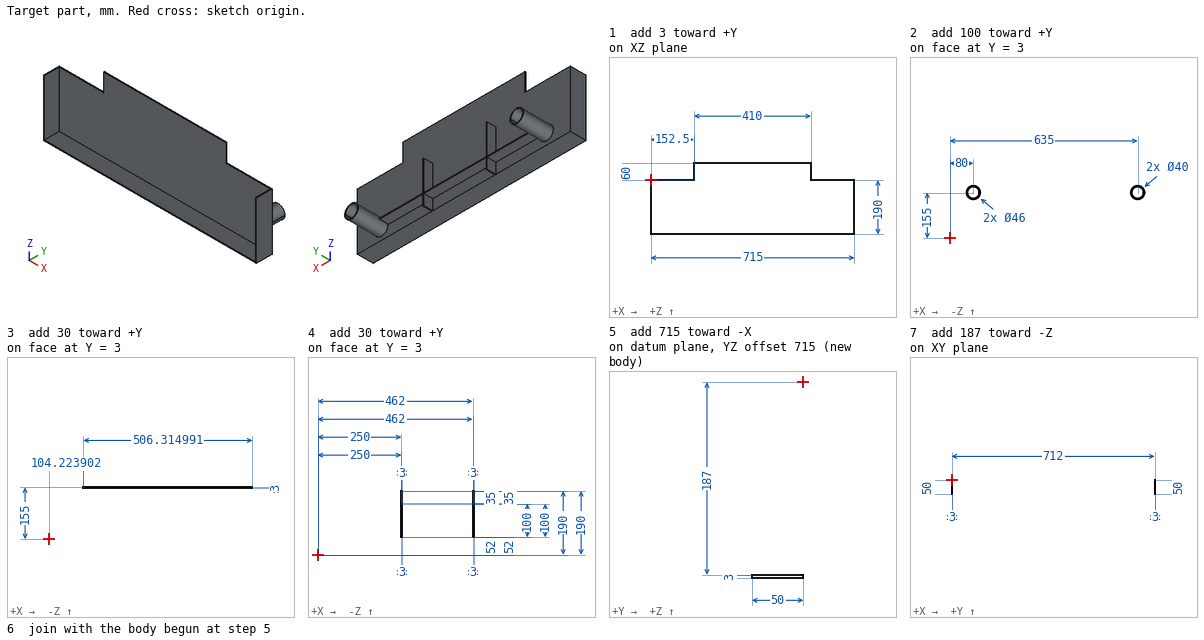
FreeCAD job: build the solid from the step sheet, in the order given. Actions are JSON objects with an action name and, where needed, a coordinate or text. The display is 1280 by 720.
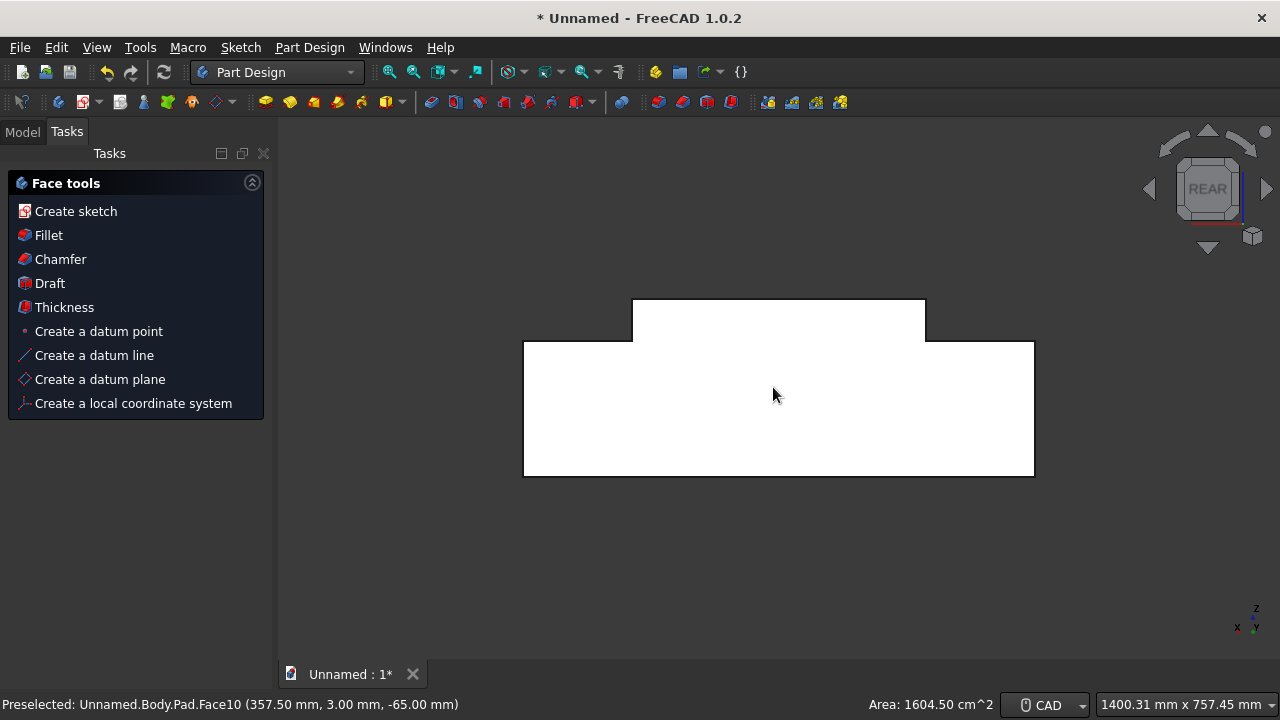
{"action": "left_click", "coordinate": [84, 102]}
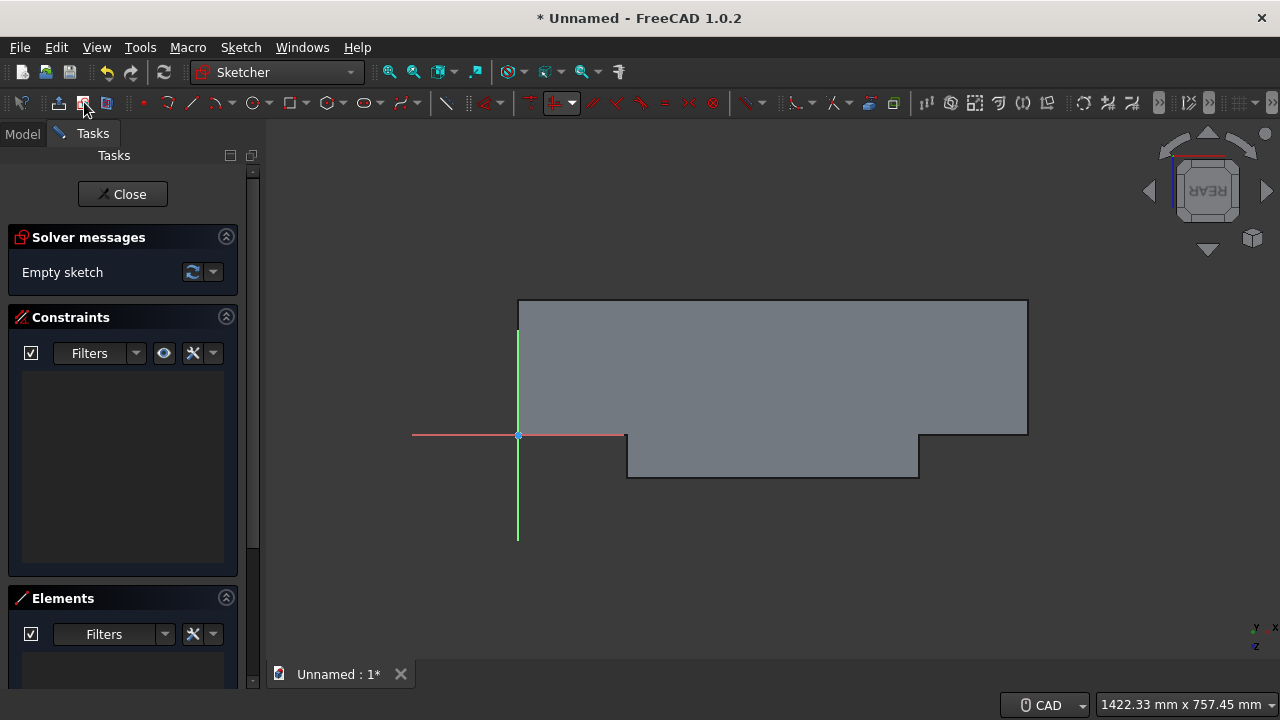
{"action": "key", "text": "g c"}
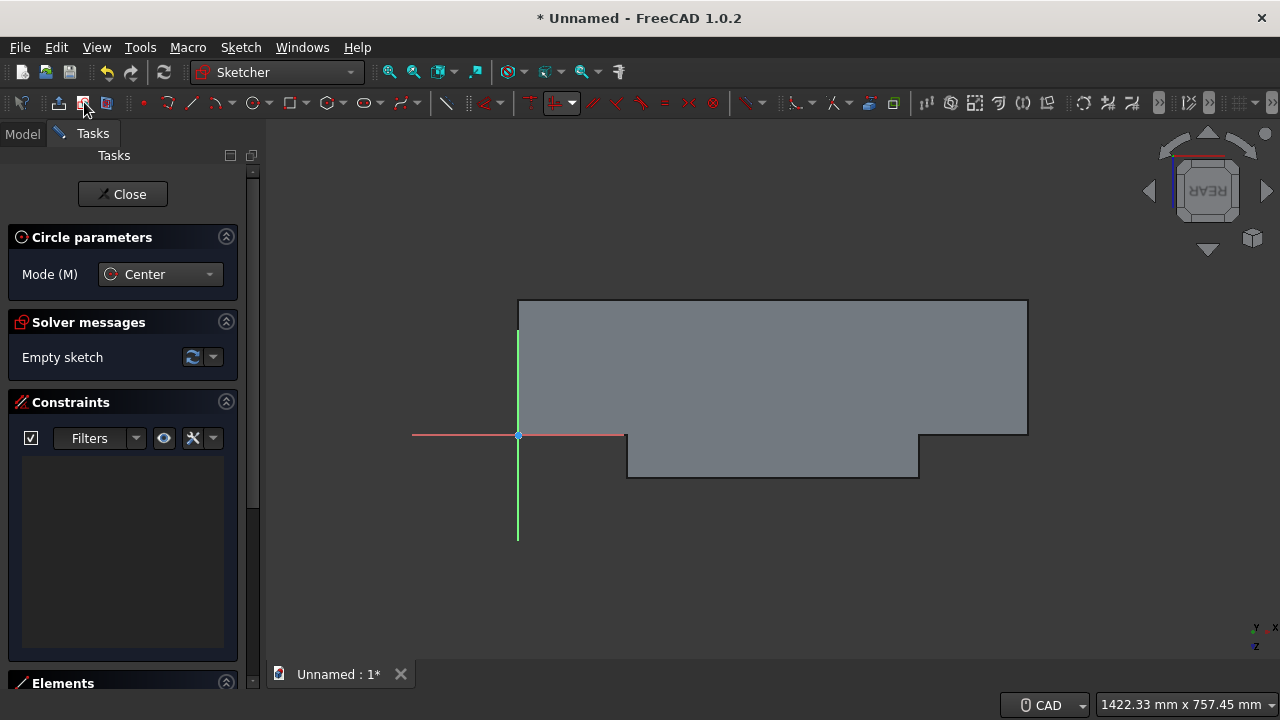
{"action": "scroll", "coordinate": [575, 325], "scroll_direction": "up", "scroll_amount": 2}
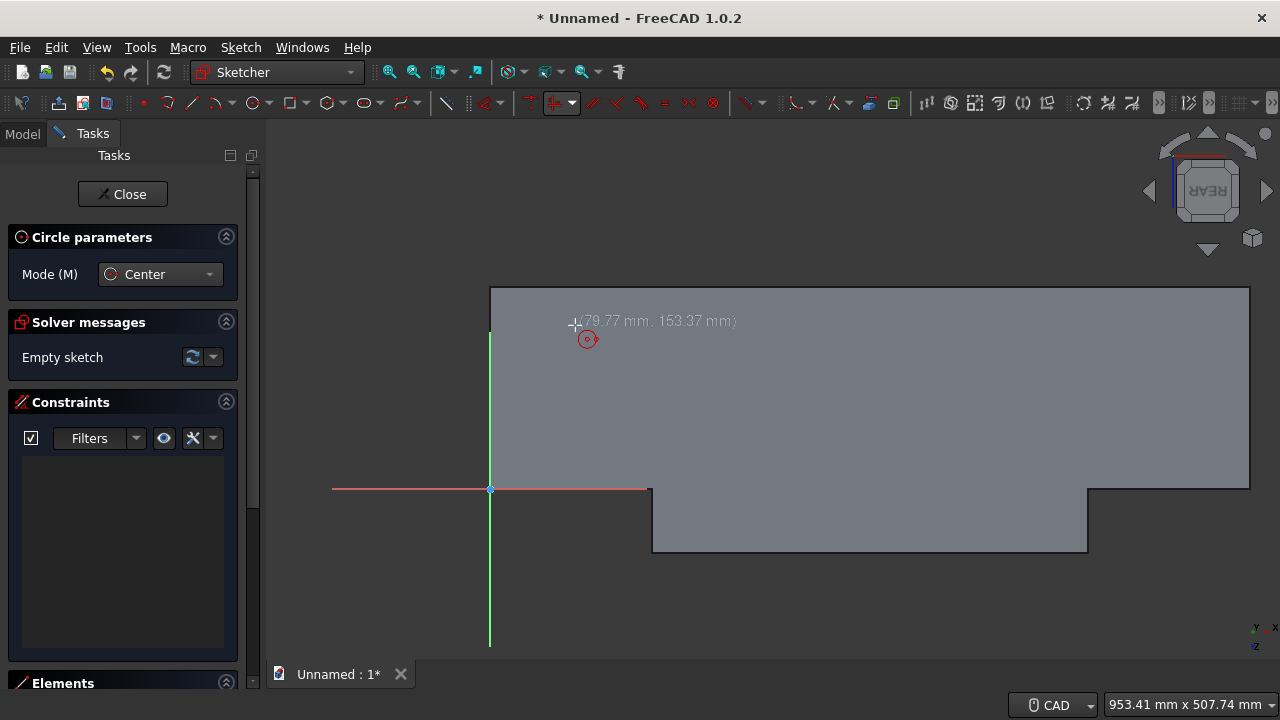
{"action": "left_click", "coordinate": [575, 325]}
{"action": "mouse_move", "coordinate": [592, 307]}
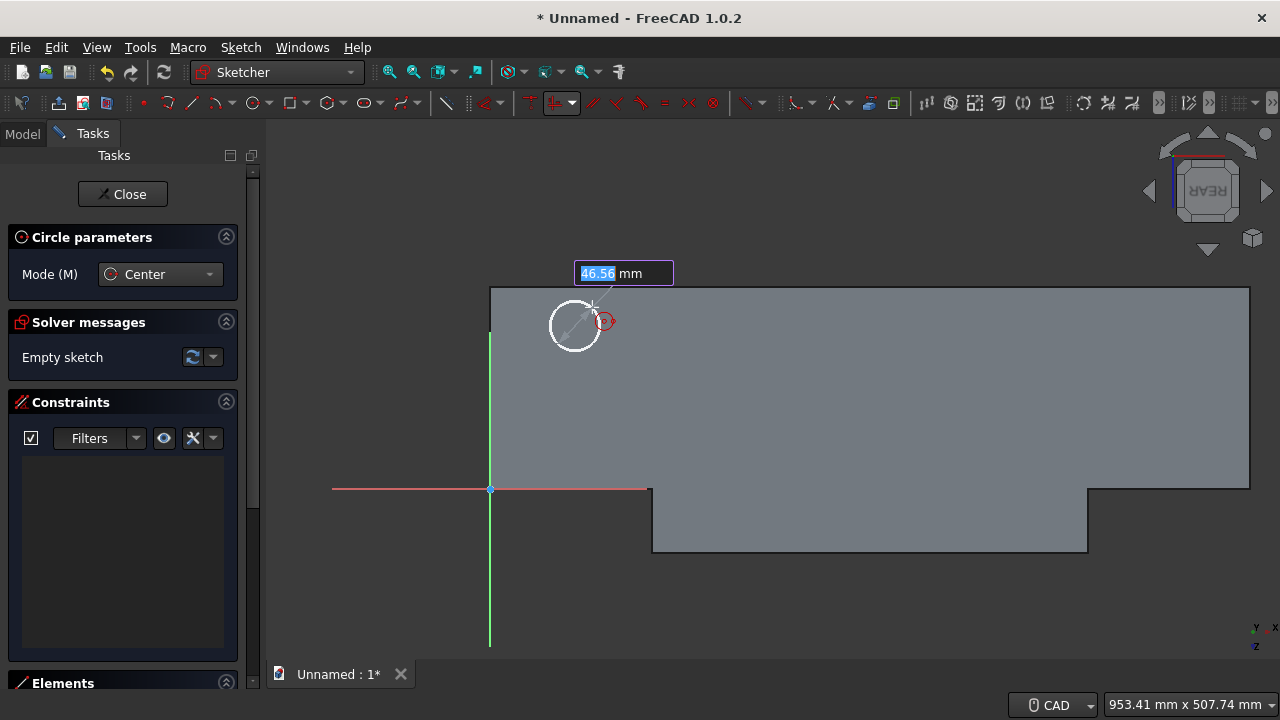
{"action": "type", "text": "46"}
{"action": "key", "text": "Return"}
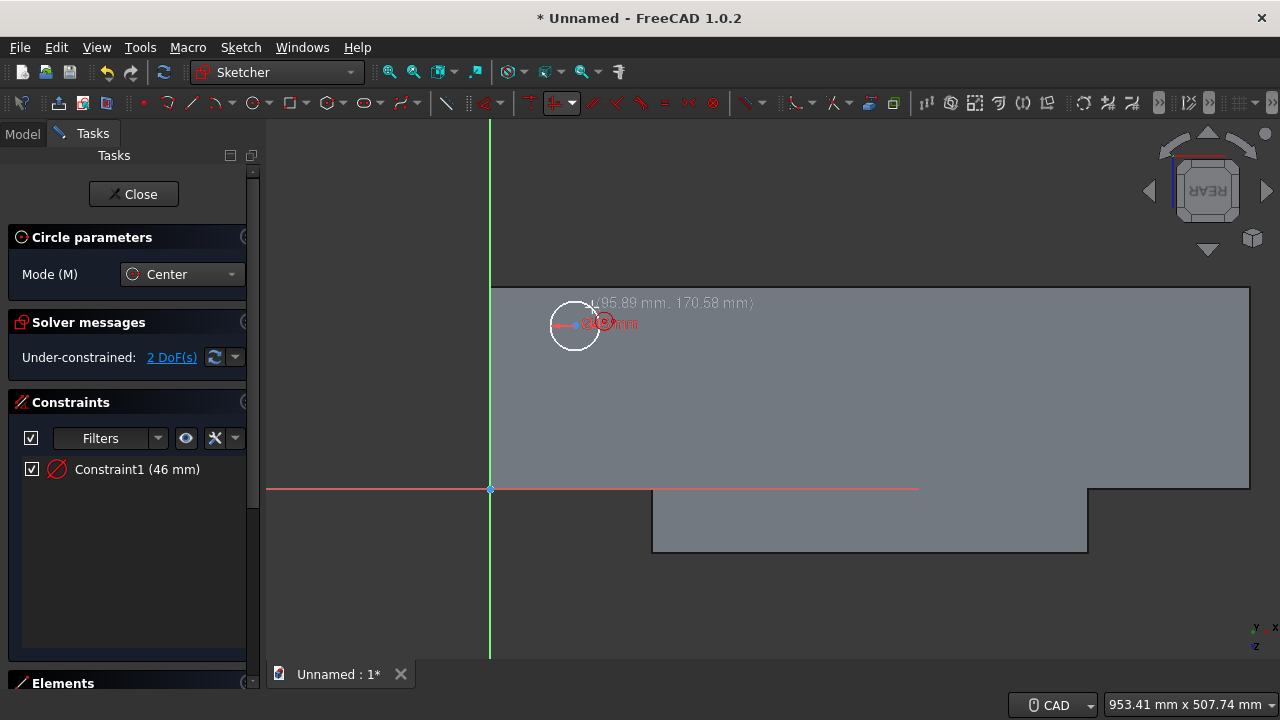
{"action": "scroll", "coordinate": [294, 363], "scroll_direction": "down", "scroll_amount": 1}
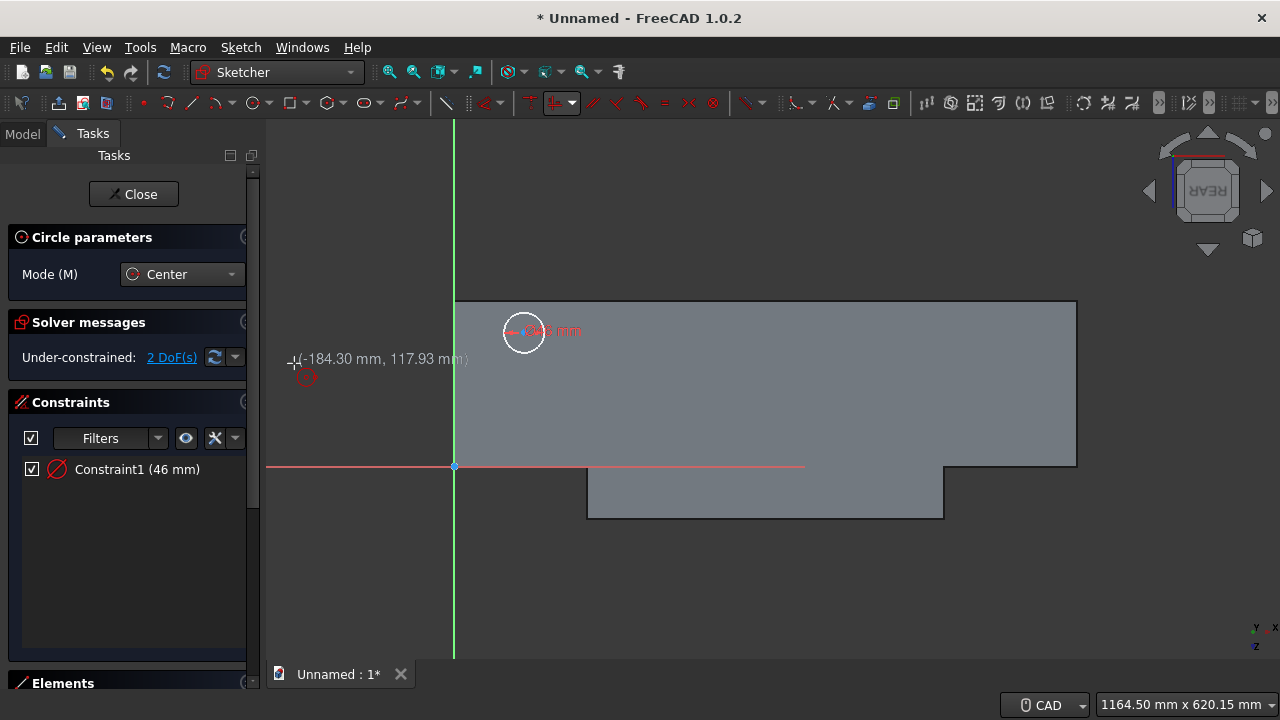
{"action": "left_click", "coordinate": [1007, 332]}
{"action": "mouse_move", "coordinate": [1022, 317]}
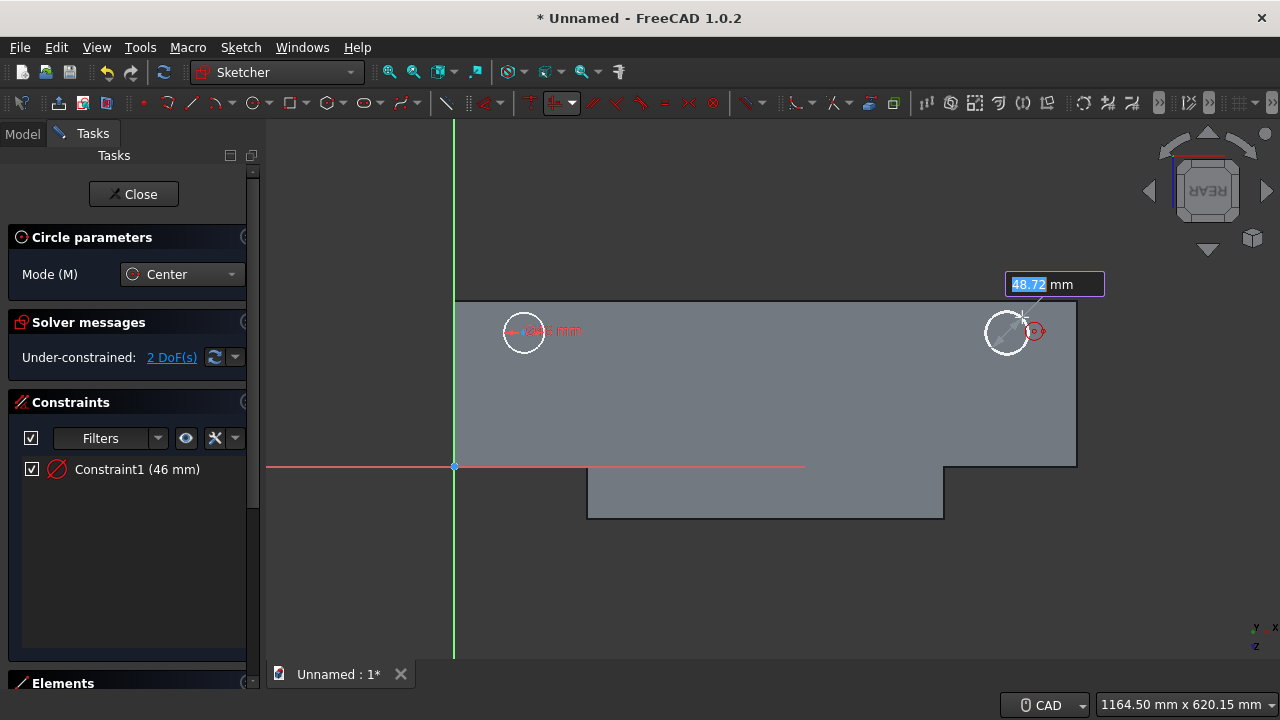
{"action": "type", "text": "46"}
{"action": "key", "text": "Return"}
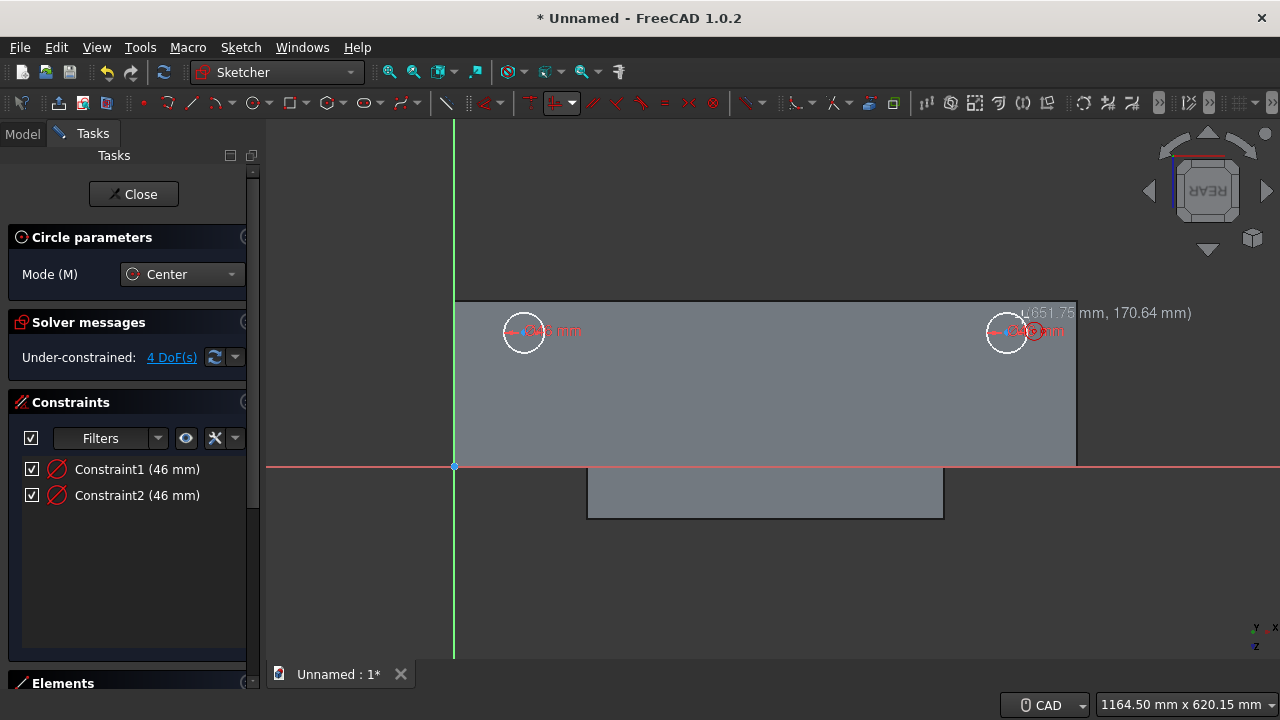
{"action": "scroll", "coordinate": [524, 332], "scroll_direction": "up", "scroll_amount": 2}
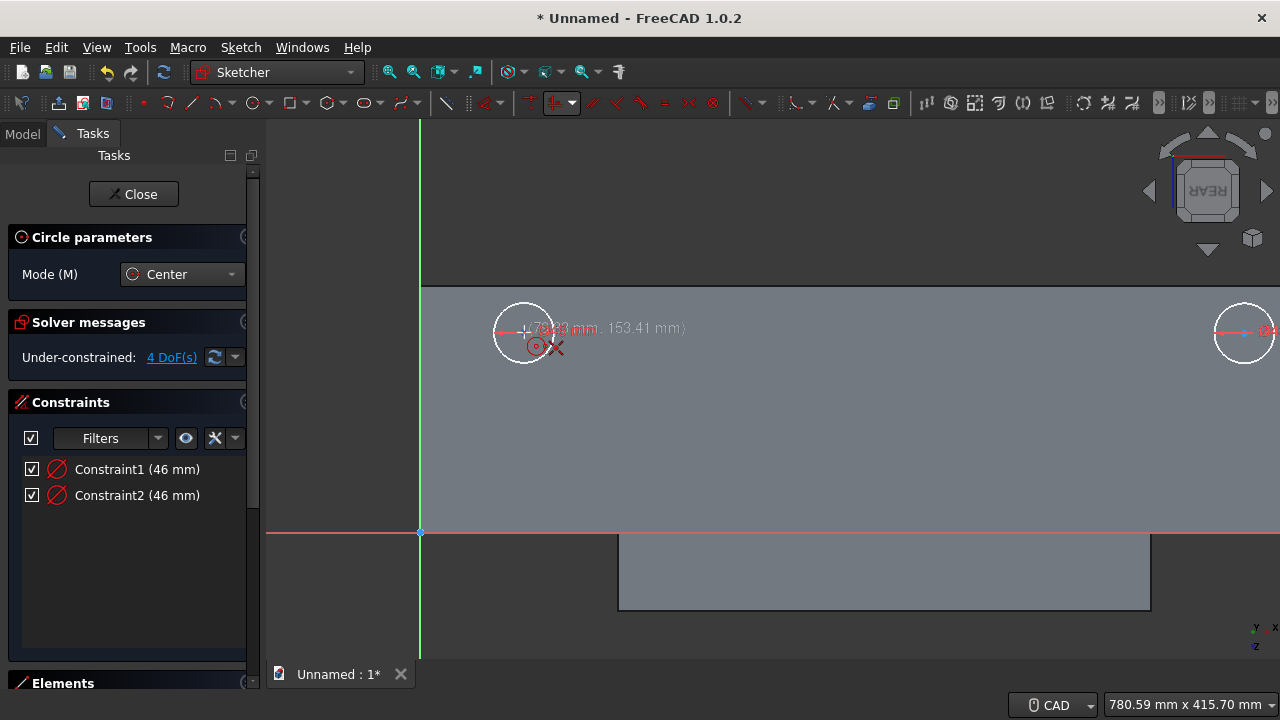
{"action": "left_click", "coordinate": [524, 333]}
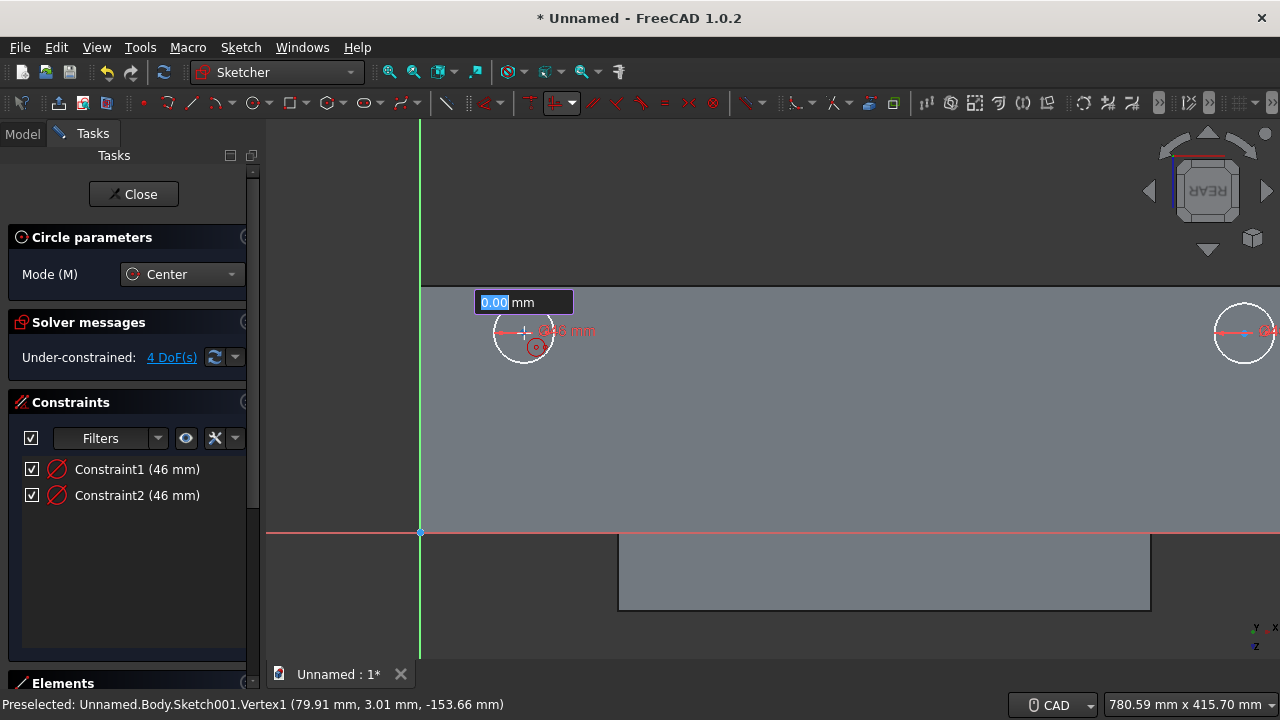
{"action": "scroll", "coordinate": [533, 307], "scroll_direction": "up", "scroll_amount": 8}
{"action": "mouse_move", "coordinate": [532, 305]}